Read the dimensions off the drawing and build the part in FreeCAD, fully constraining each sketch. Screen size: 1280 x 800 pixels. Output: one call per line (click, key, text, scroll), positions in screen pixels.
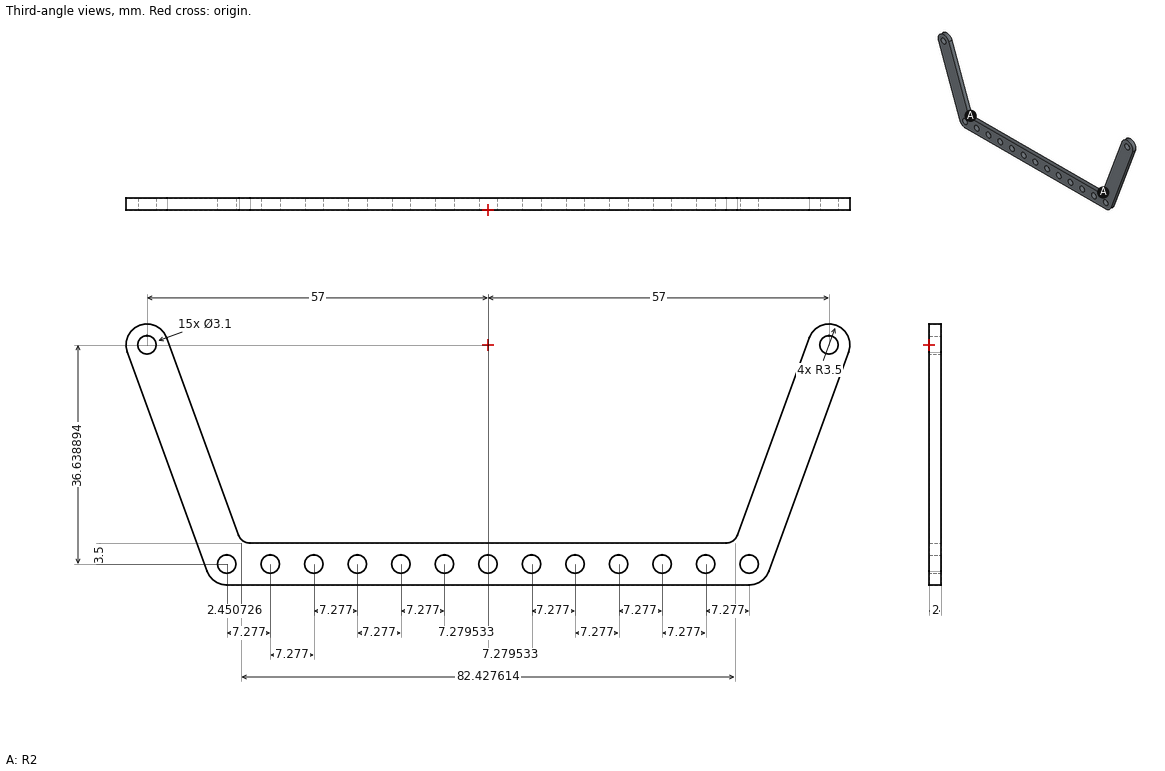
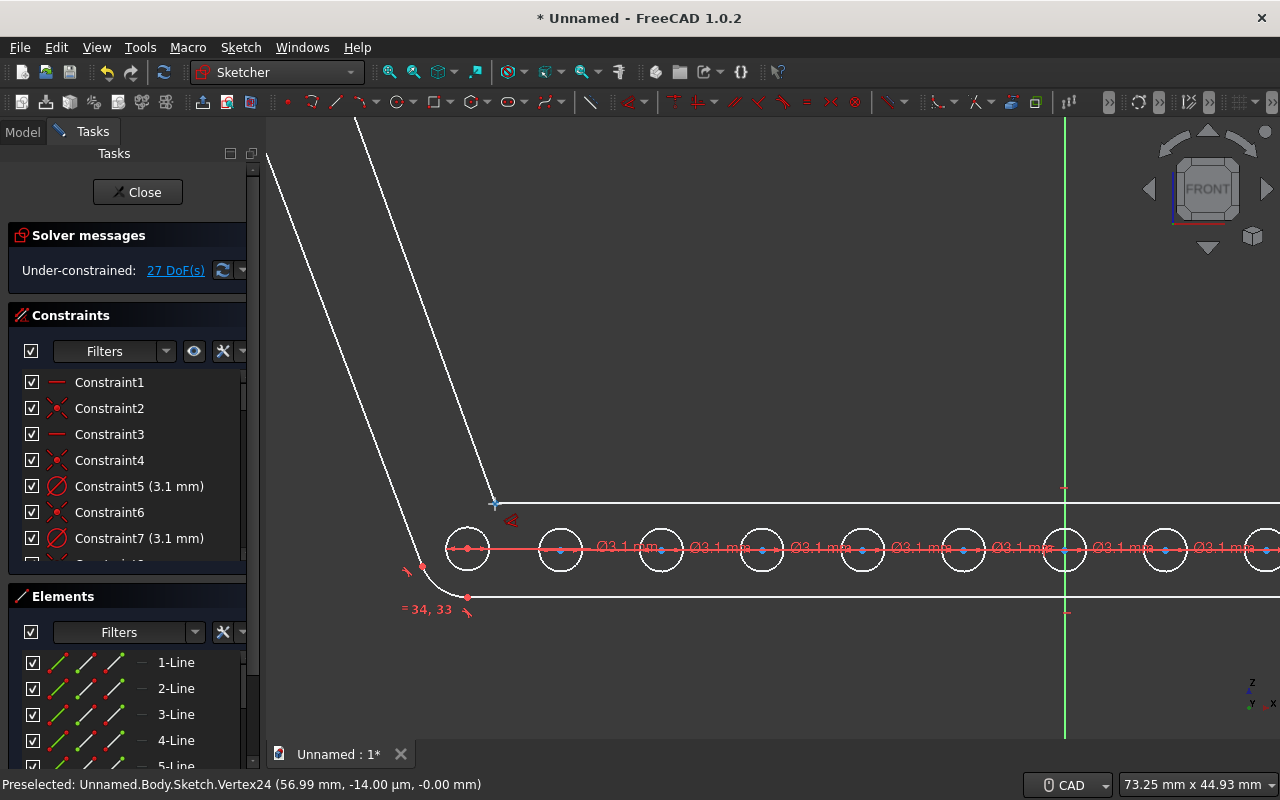
click(495, 503)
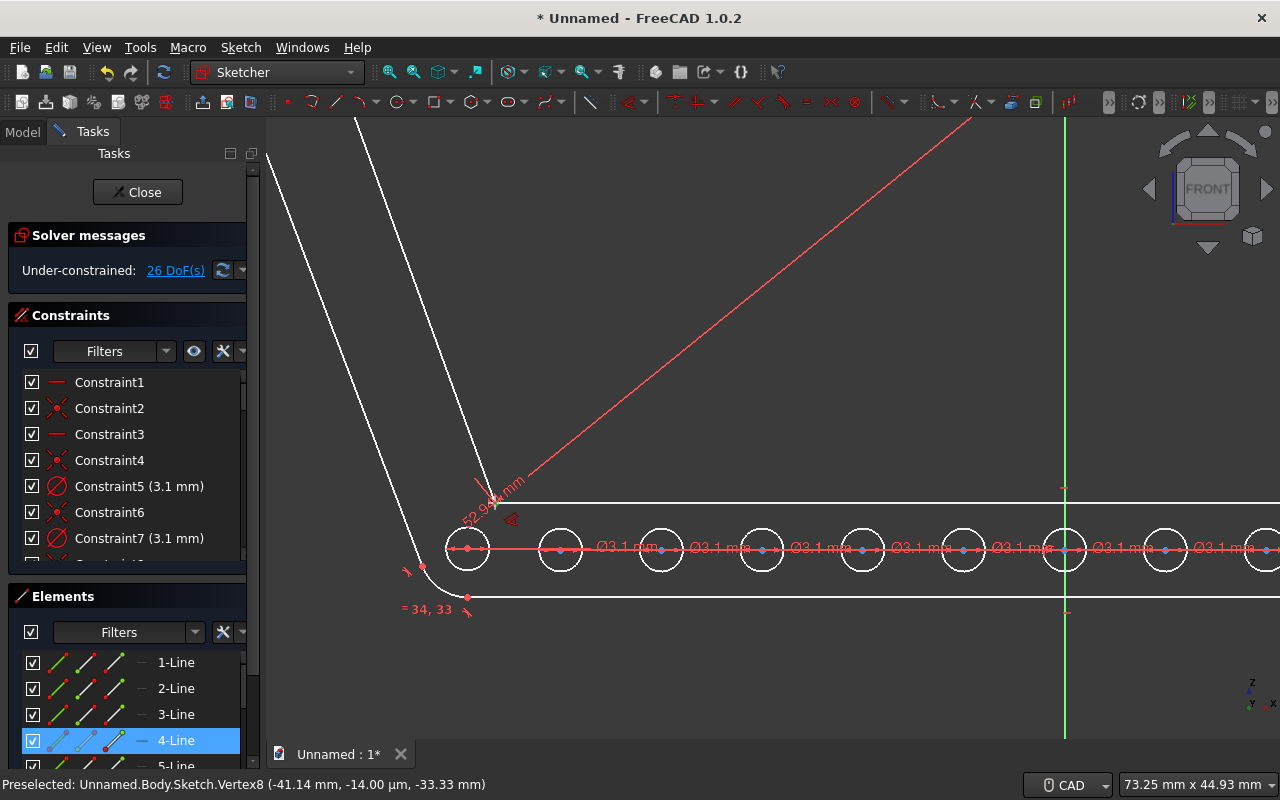
click(468, 549)
click(434, 526)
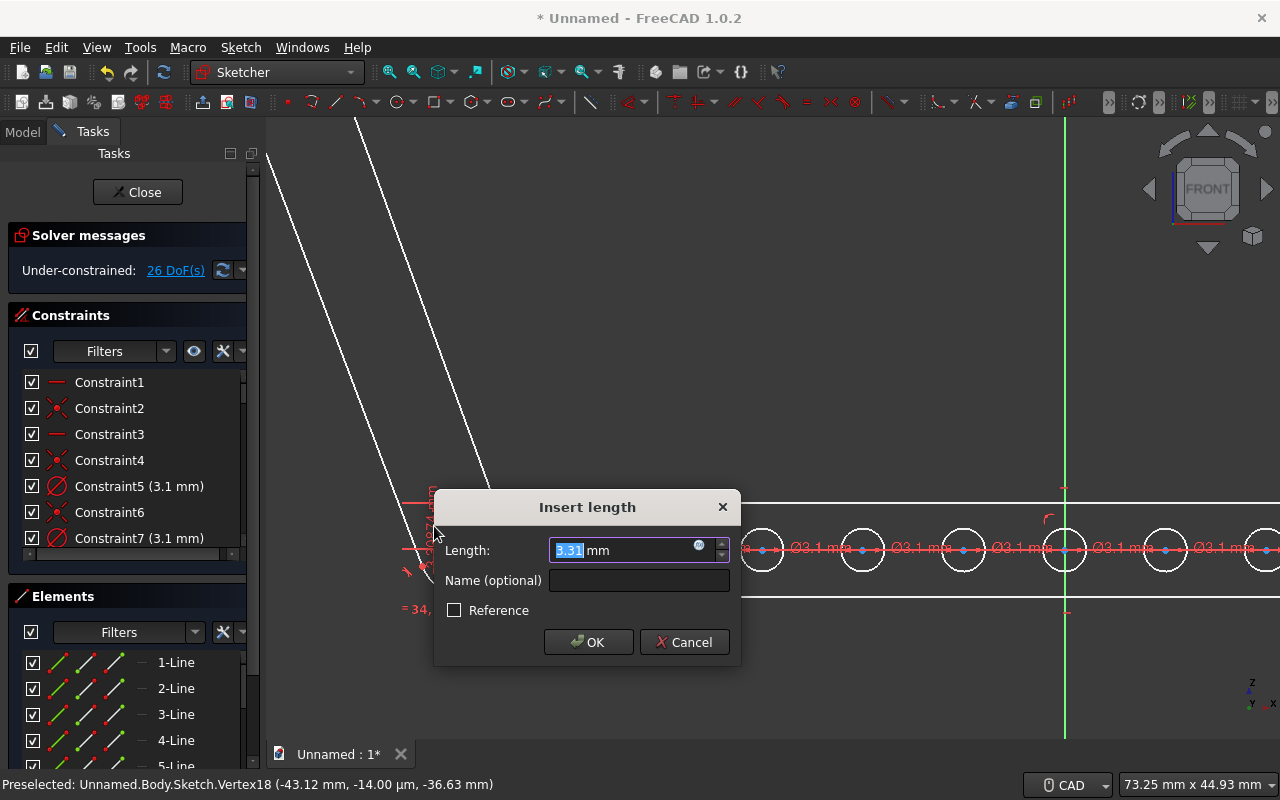
text(3.5)
key(Return)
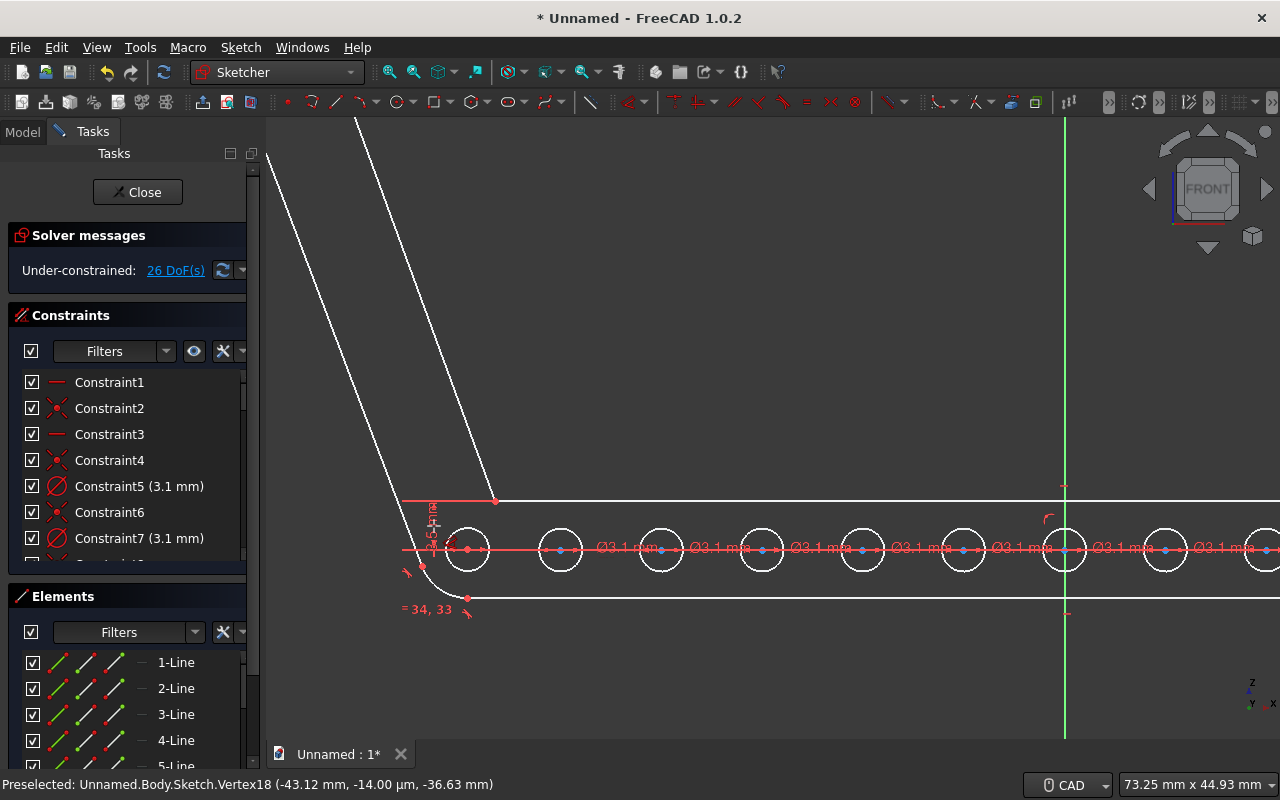
click(495, 501)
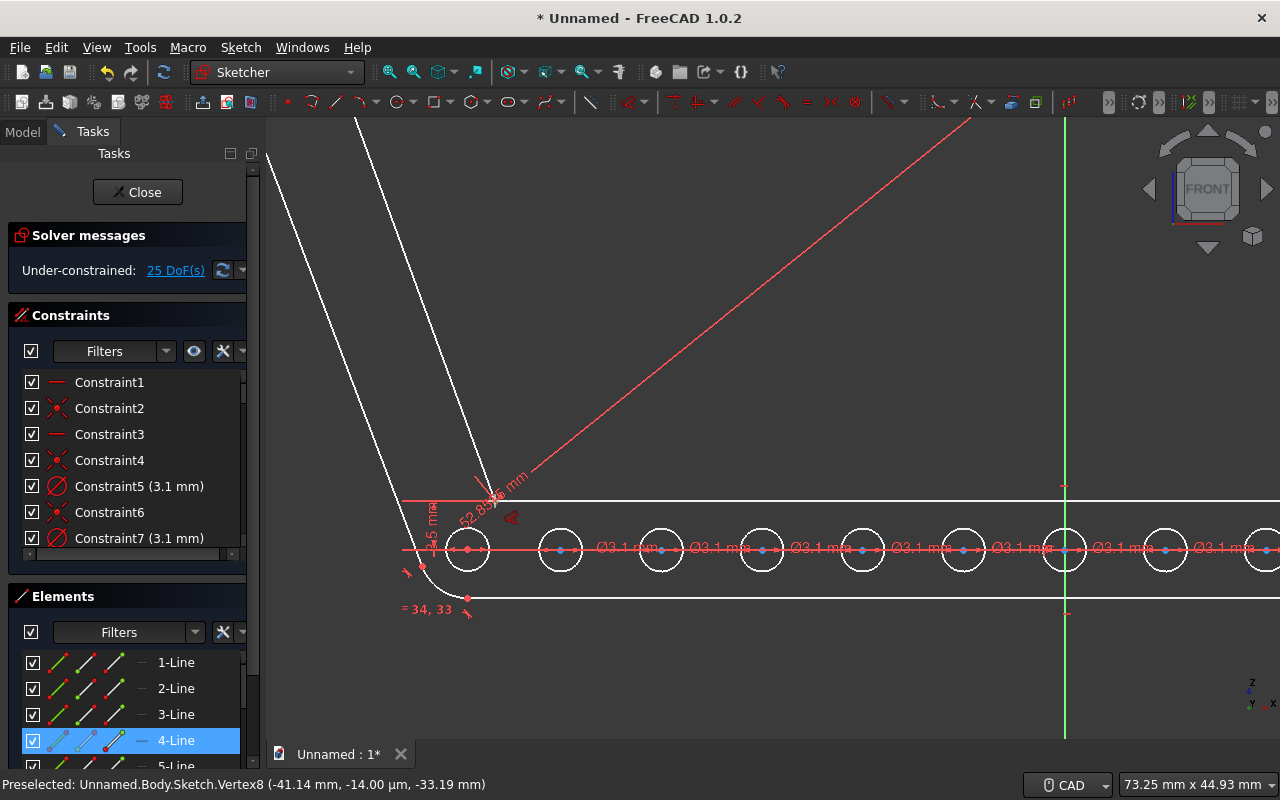
click(561, 550)
click(595, 526)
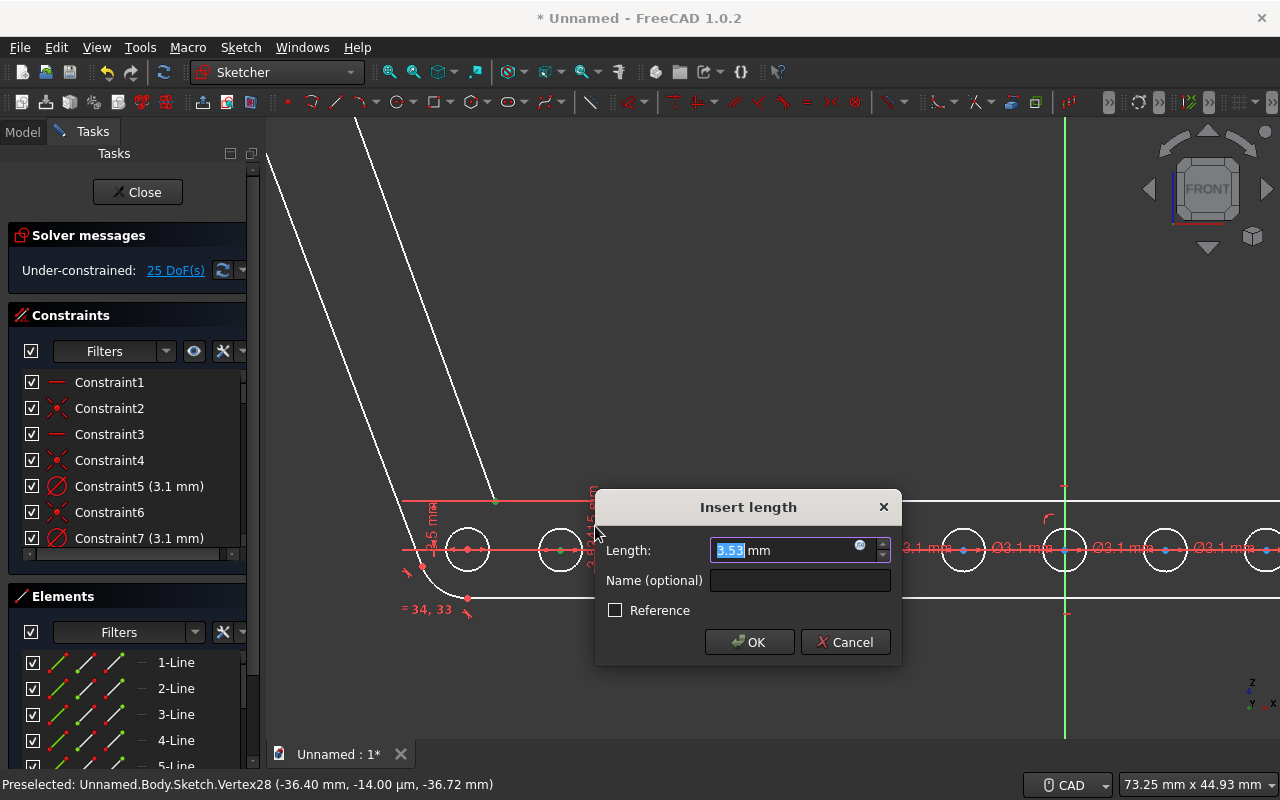
text(3.5)
key(Return)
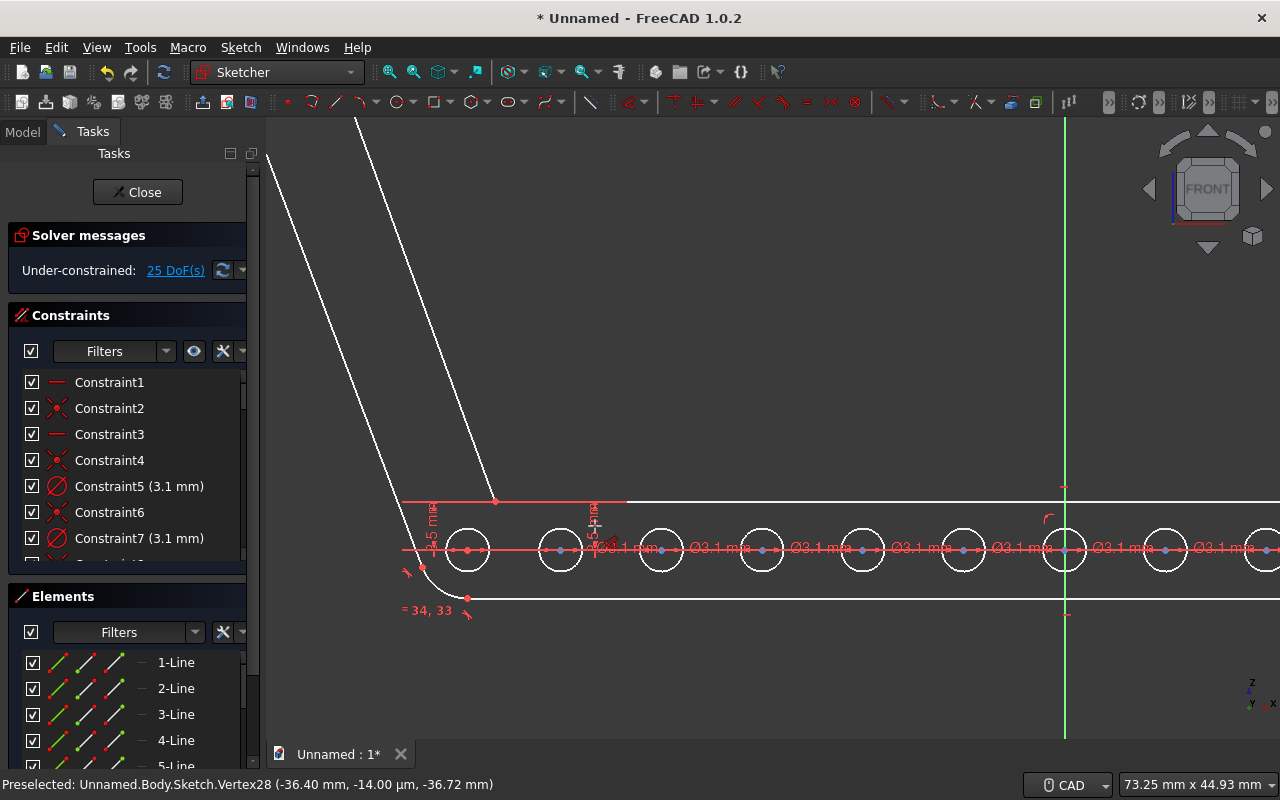
click(495, 502)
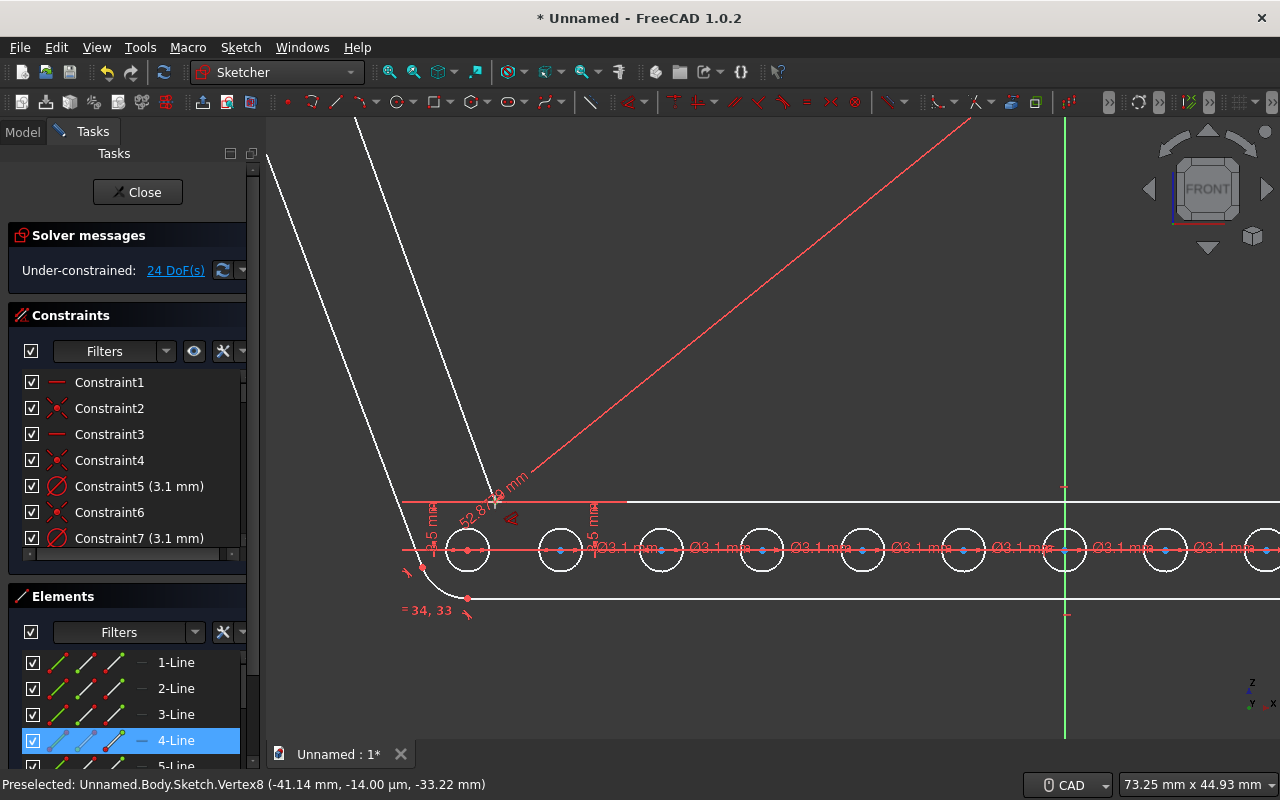
click(661, 550)
click(695, 526)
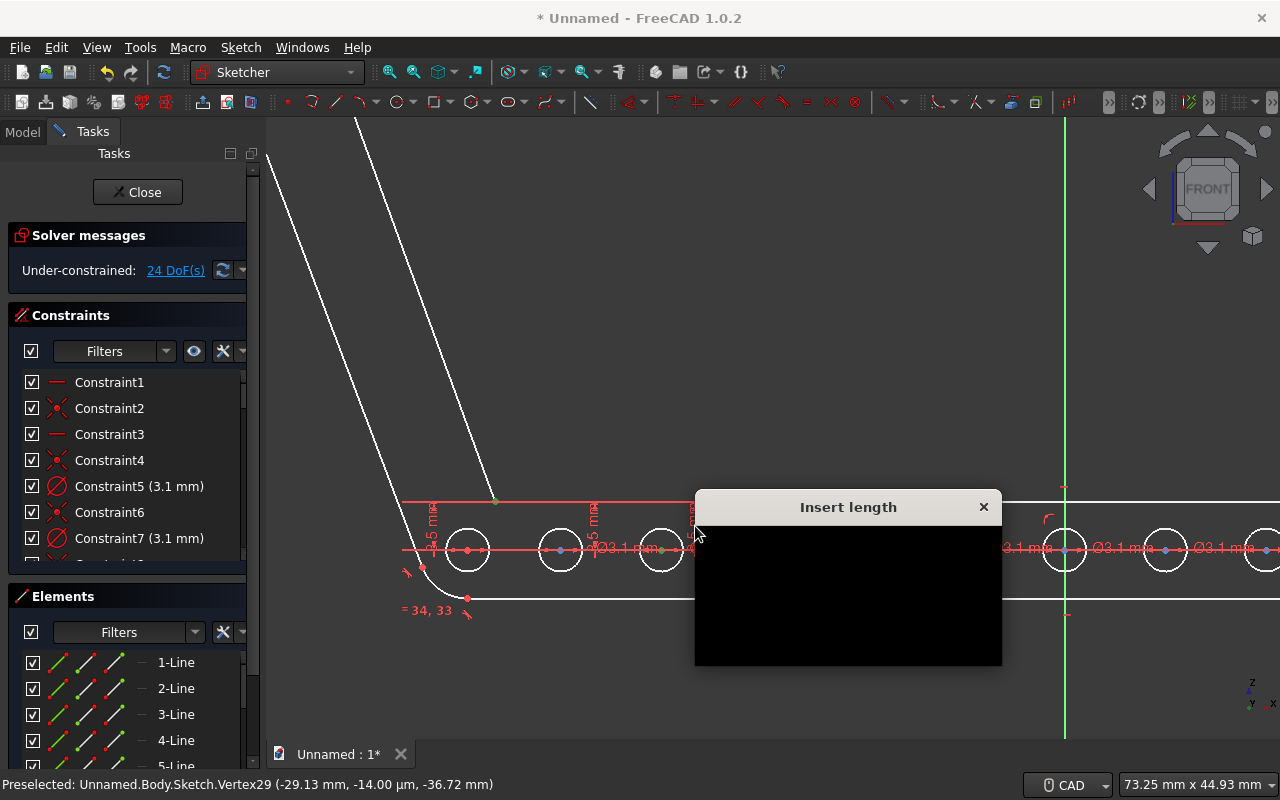
text(3.5)
key(Return)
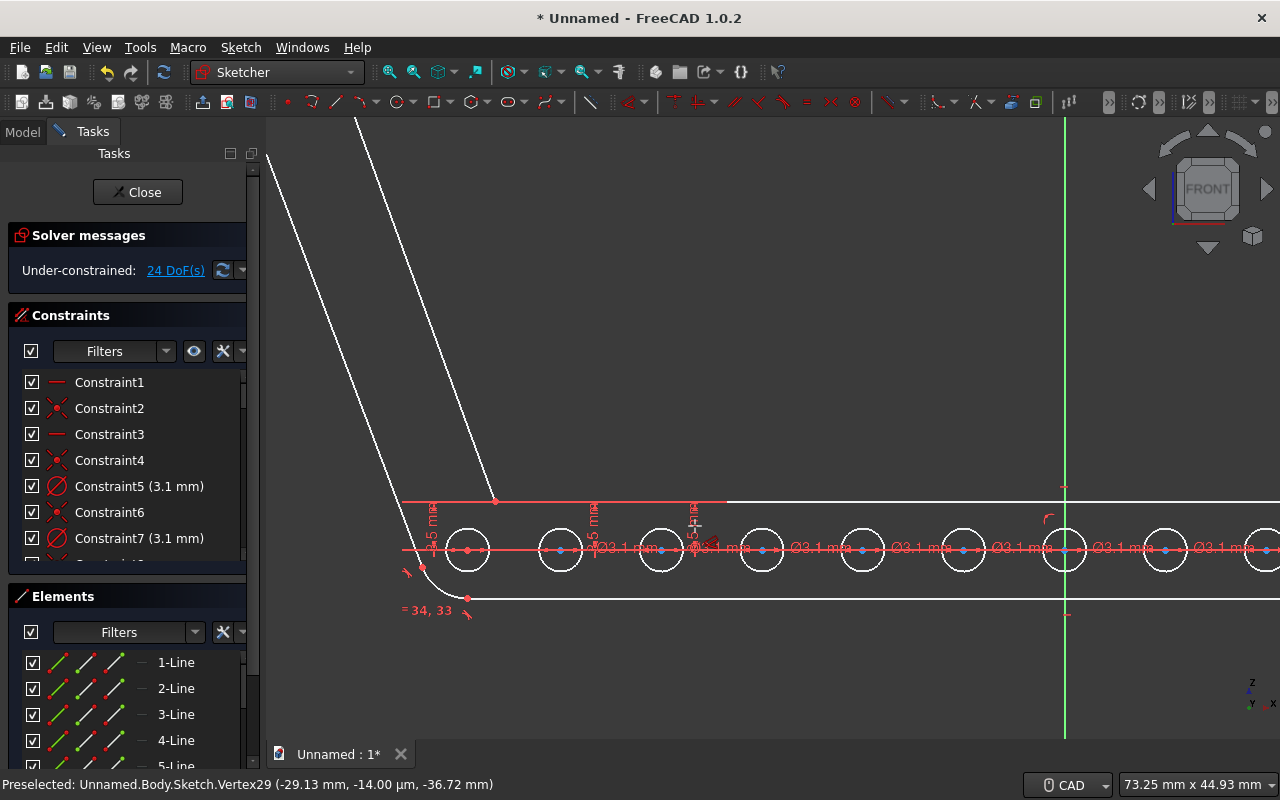
click(495, 502)